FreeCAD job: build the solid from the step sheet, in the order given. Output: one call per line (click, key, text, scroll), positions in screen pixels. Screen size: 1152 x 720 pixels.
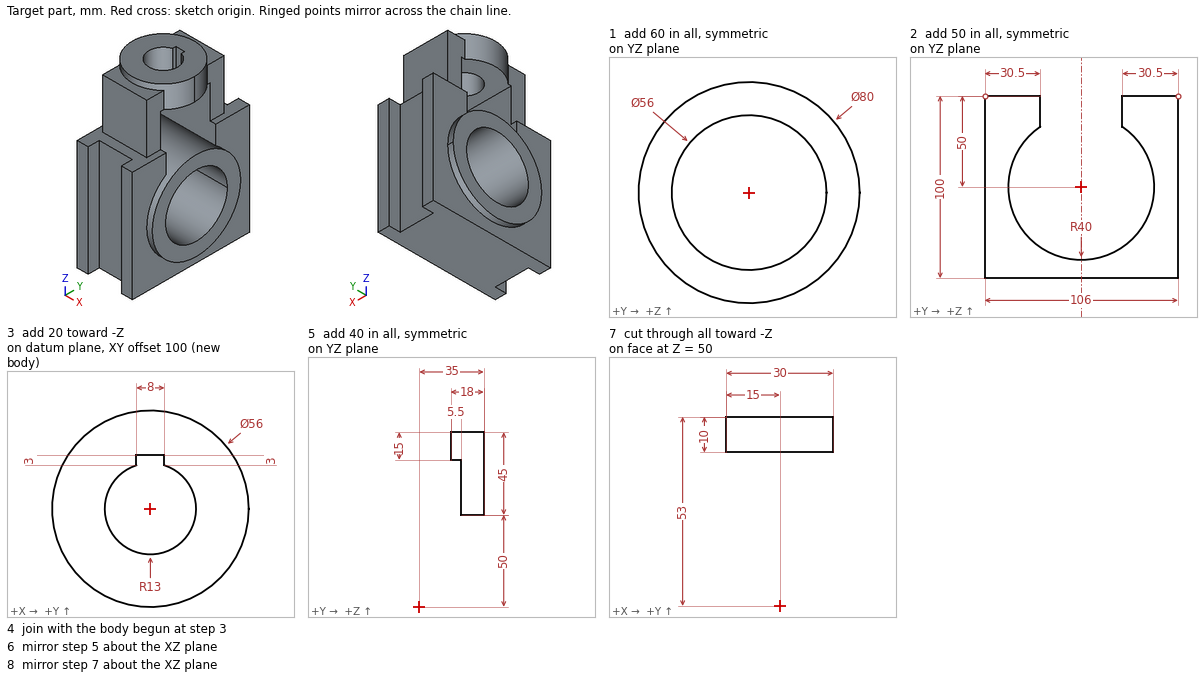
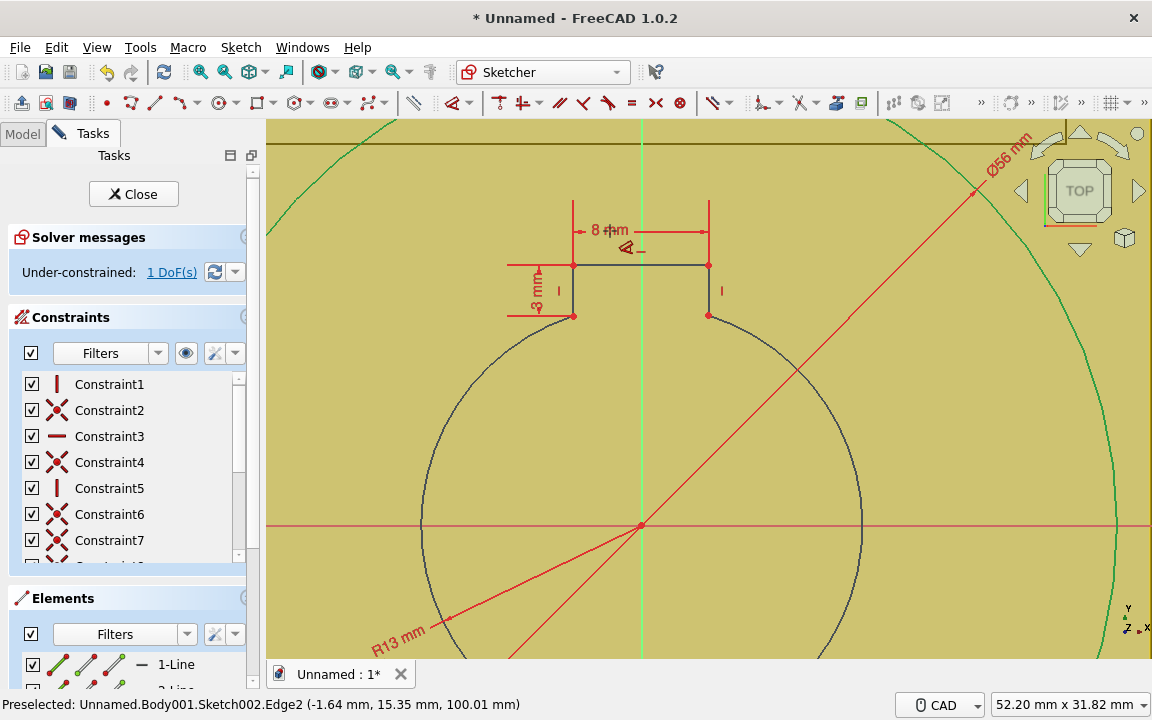
click(709, 280)
click(743, 290)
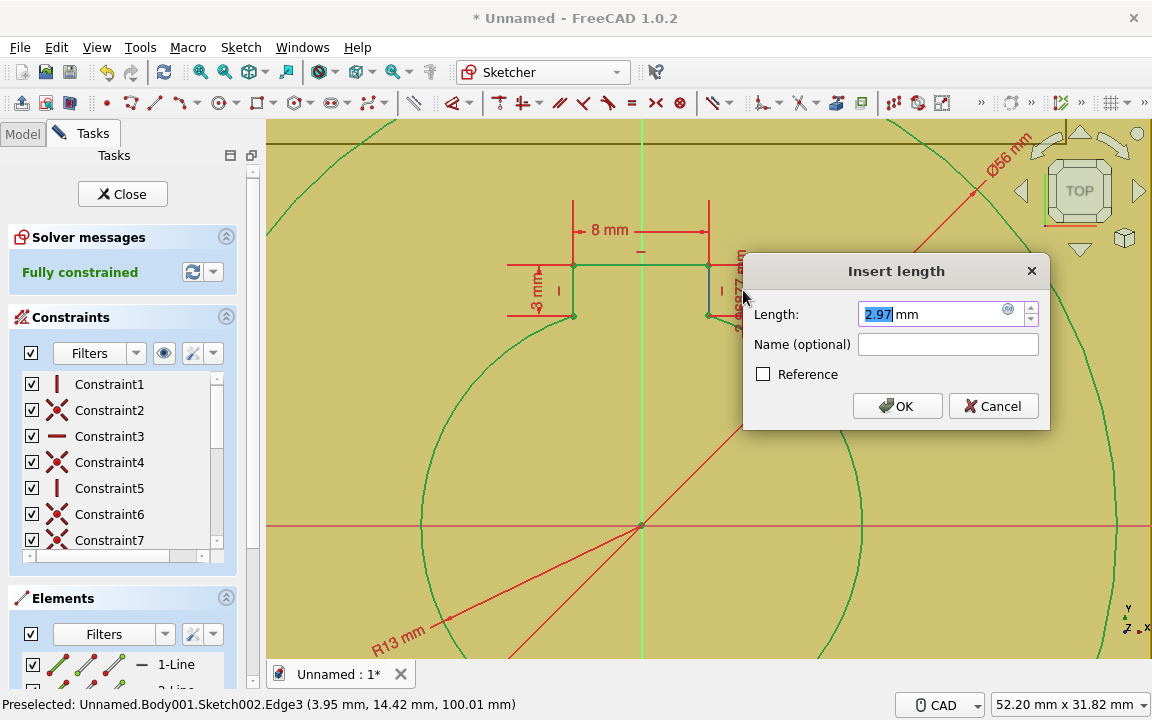
text(3)
key(Return)
key(Escape)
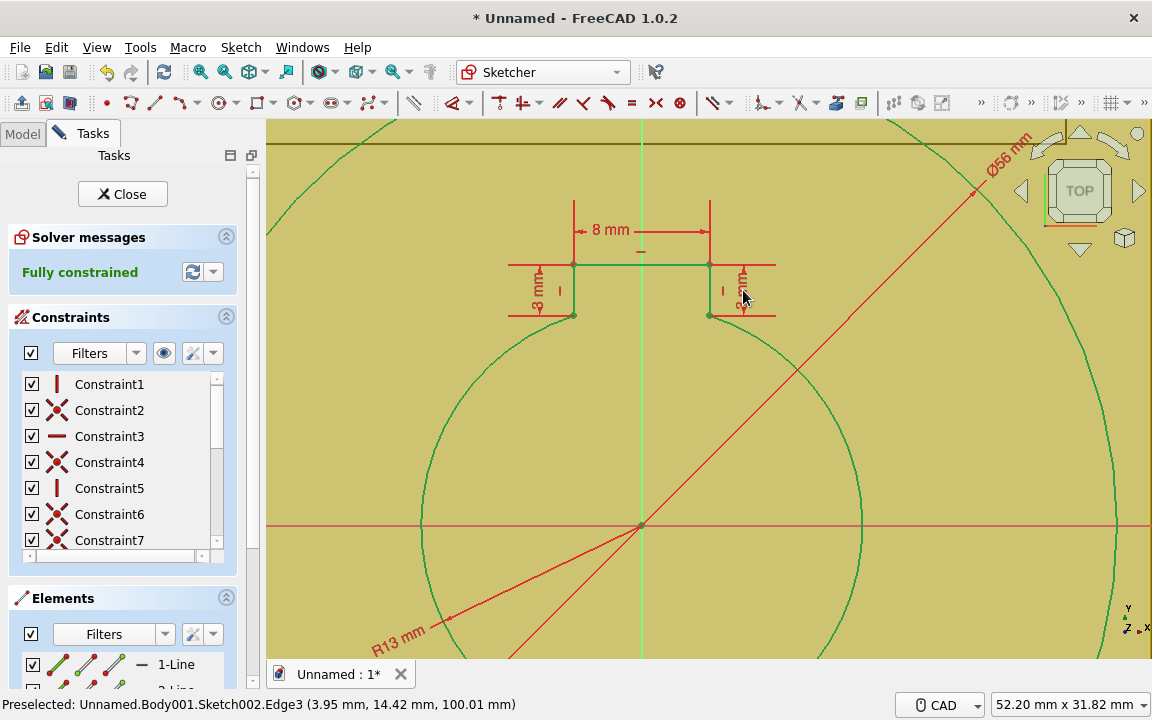
click(123, 194)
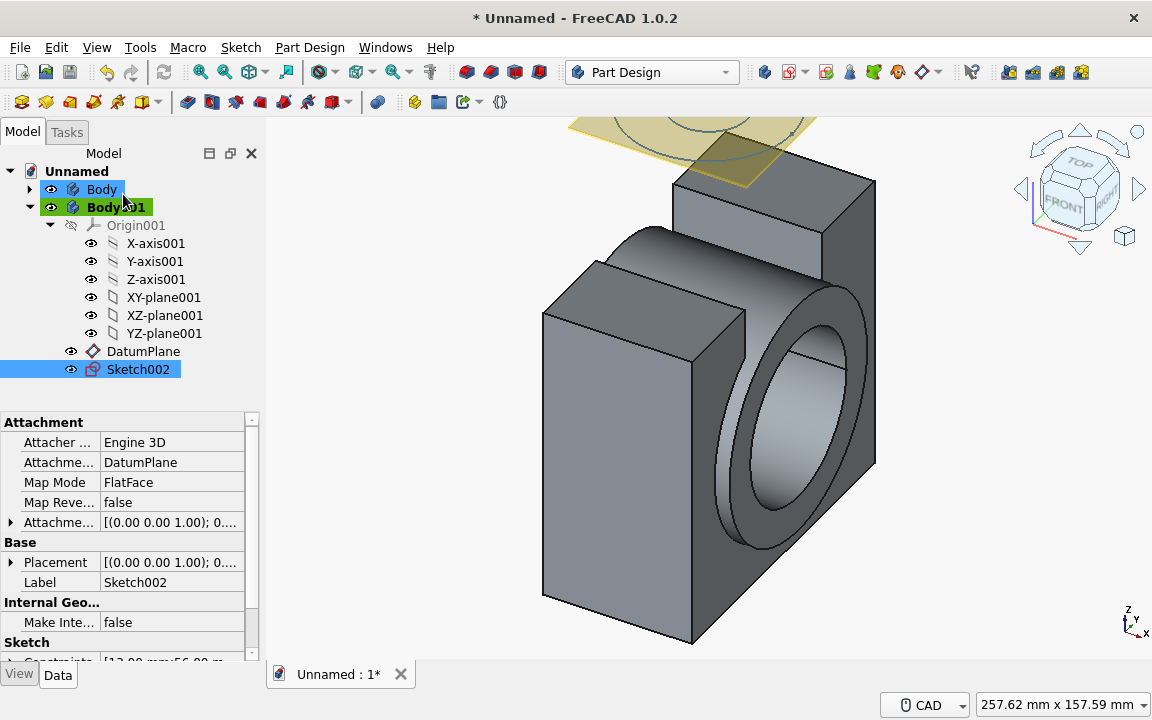
click(22, 102)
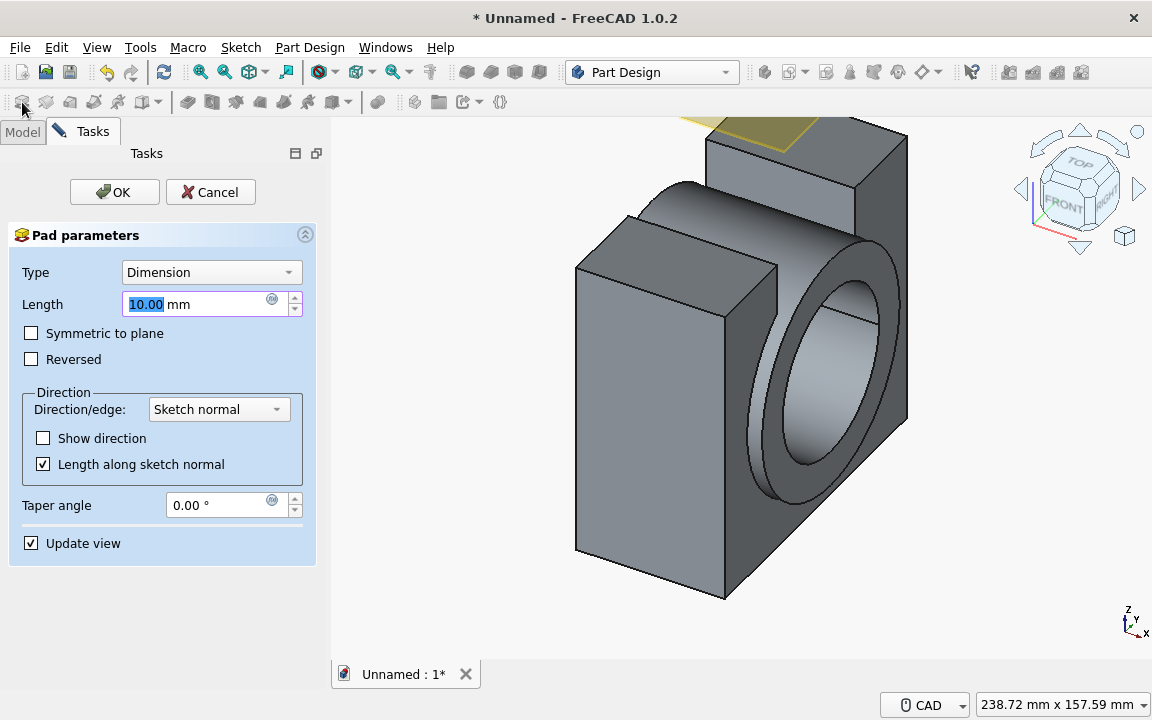
text(20)
key(Tab)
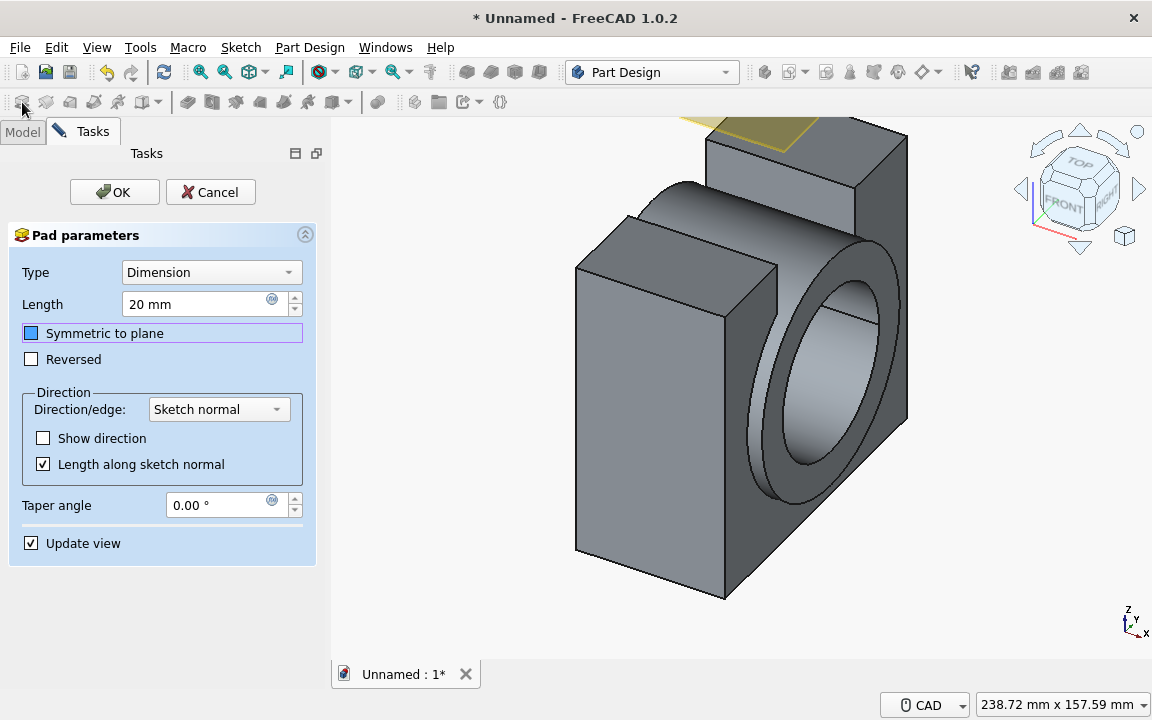
click(30, 359)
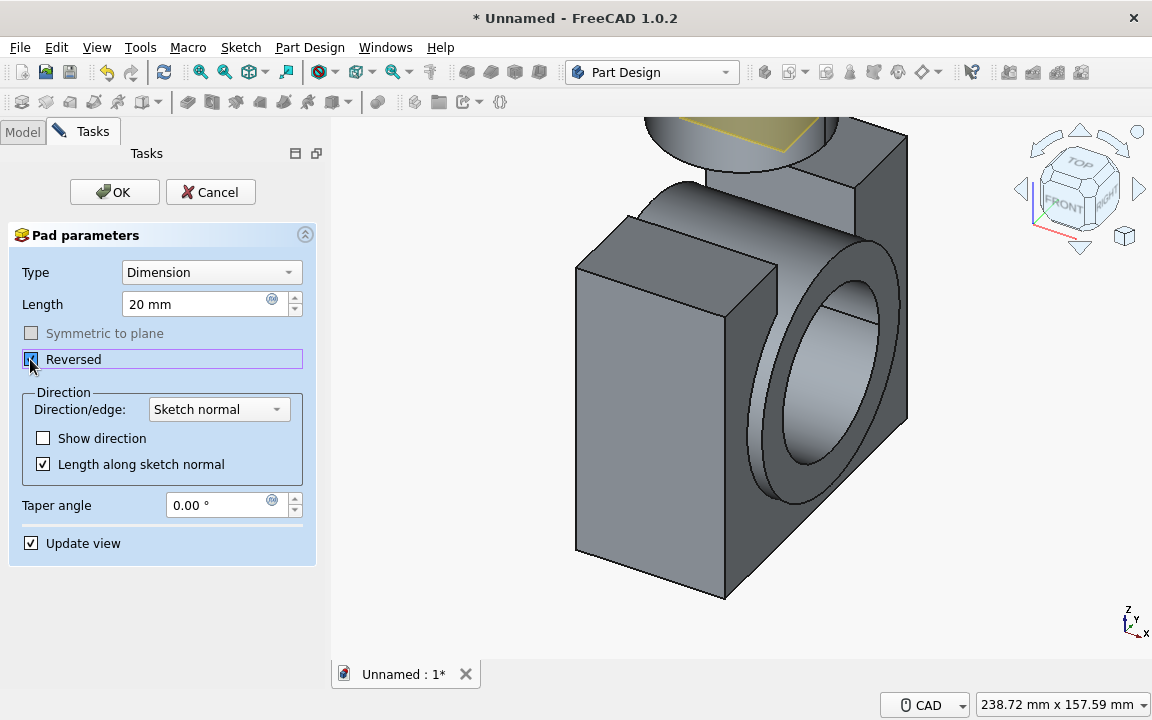
click(115, 192)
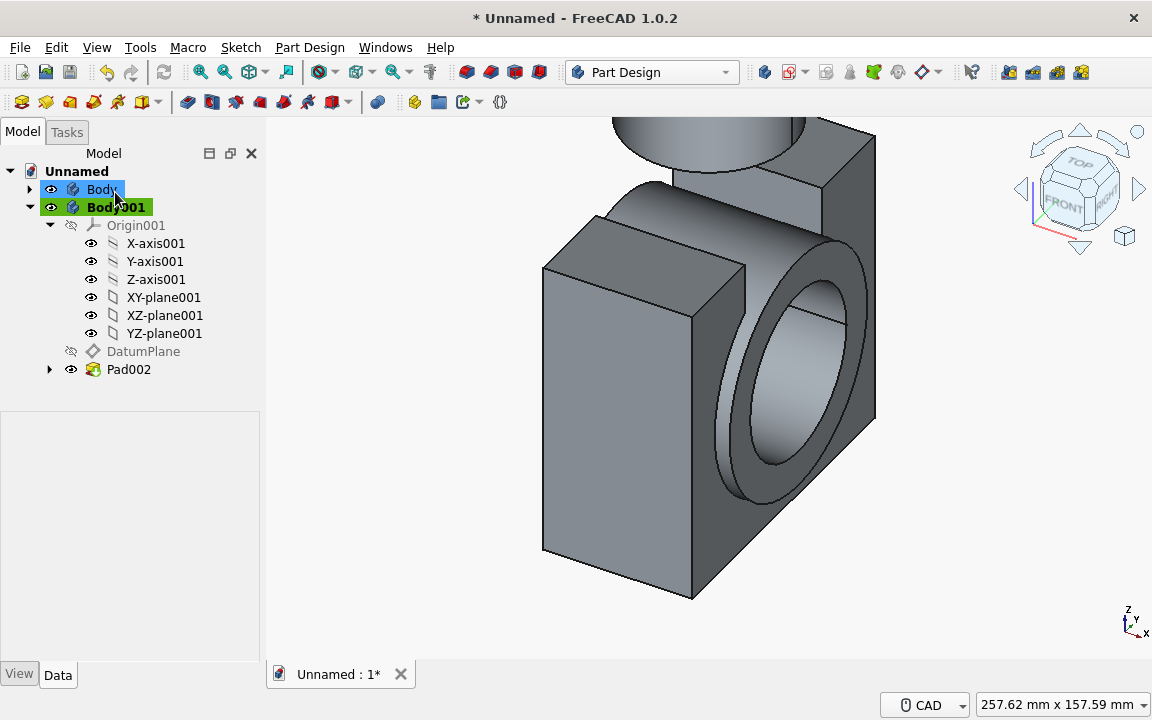
click(202, 72)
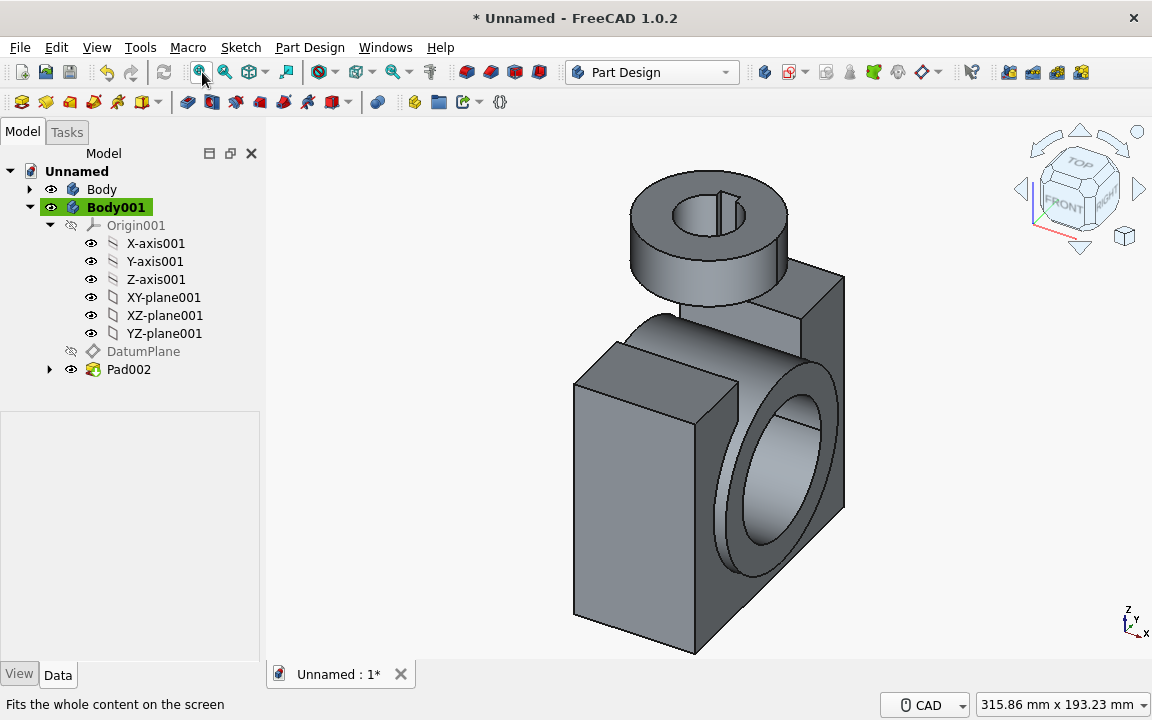
double_click(96, 189)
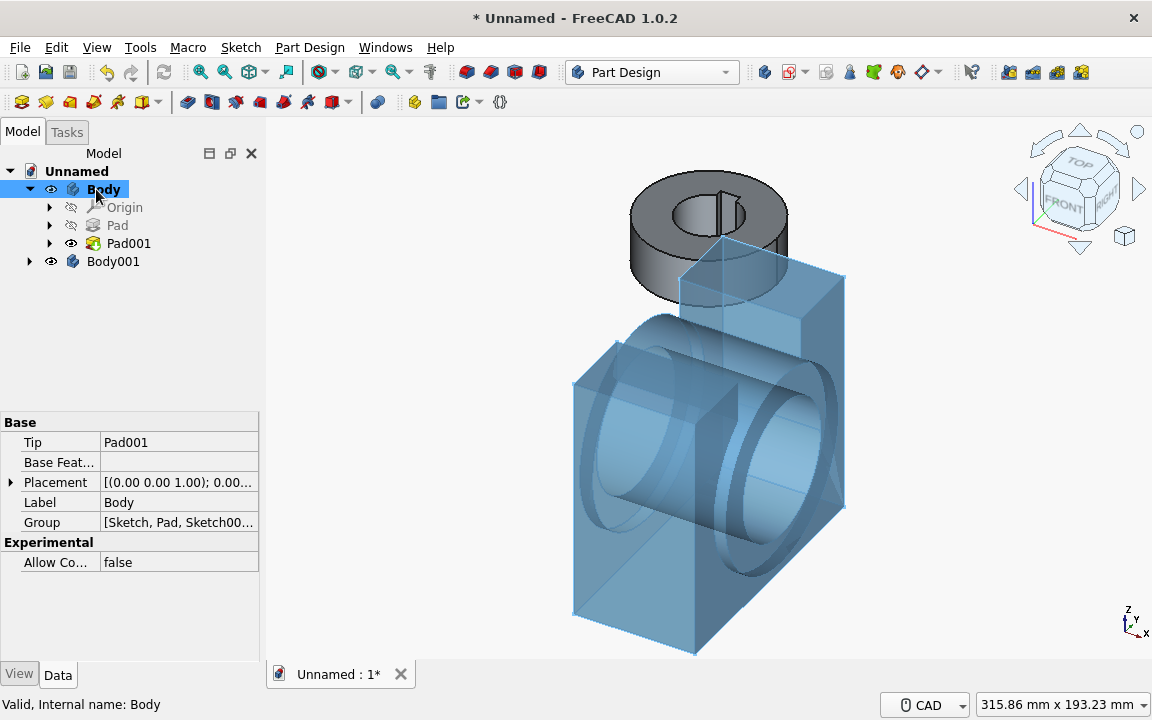
click(96, 189)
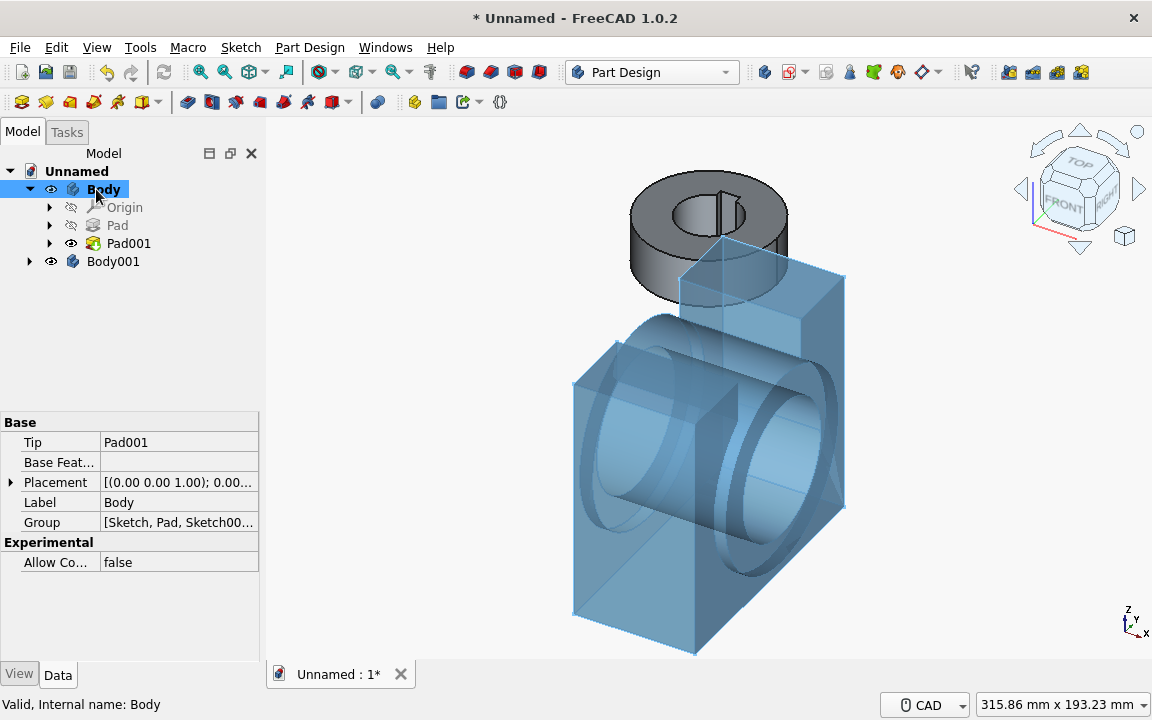
click(146, 562)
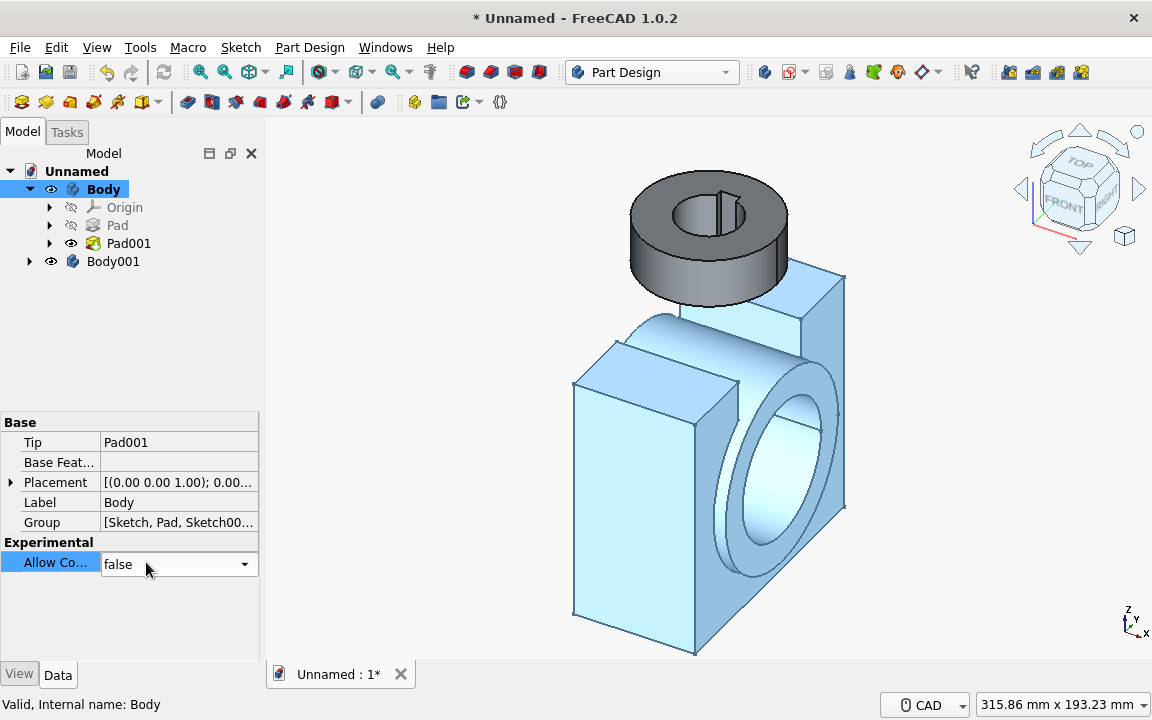
click(146, 562)